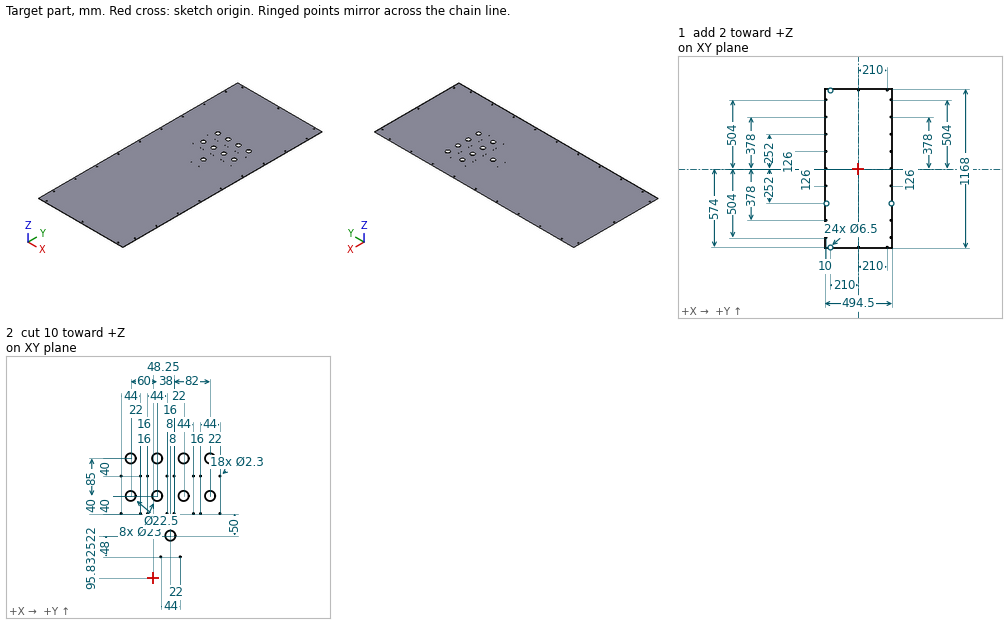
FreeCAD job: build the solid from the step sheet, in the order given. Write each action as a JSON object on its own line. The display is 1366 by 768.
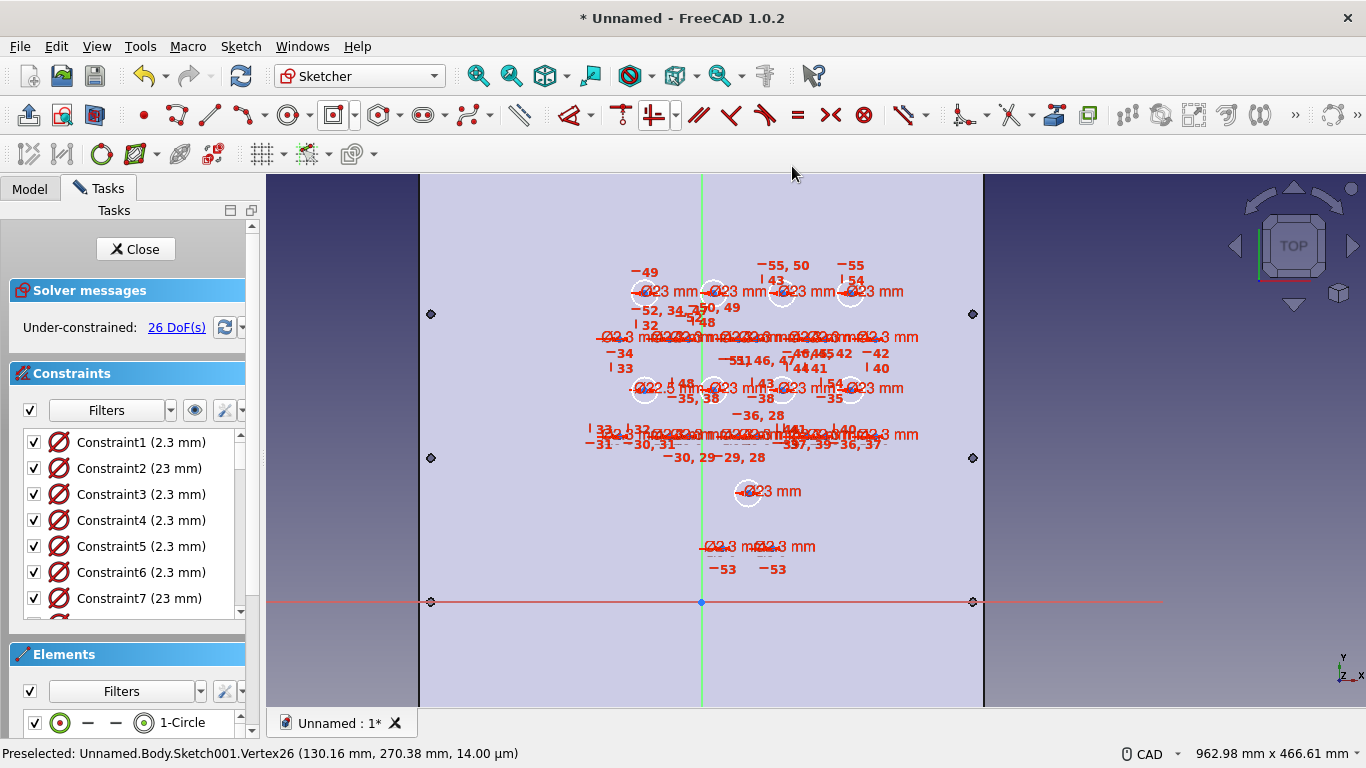
{"action": "left_click", "coordinate": [568, 116]}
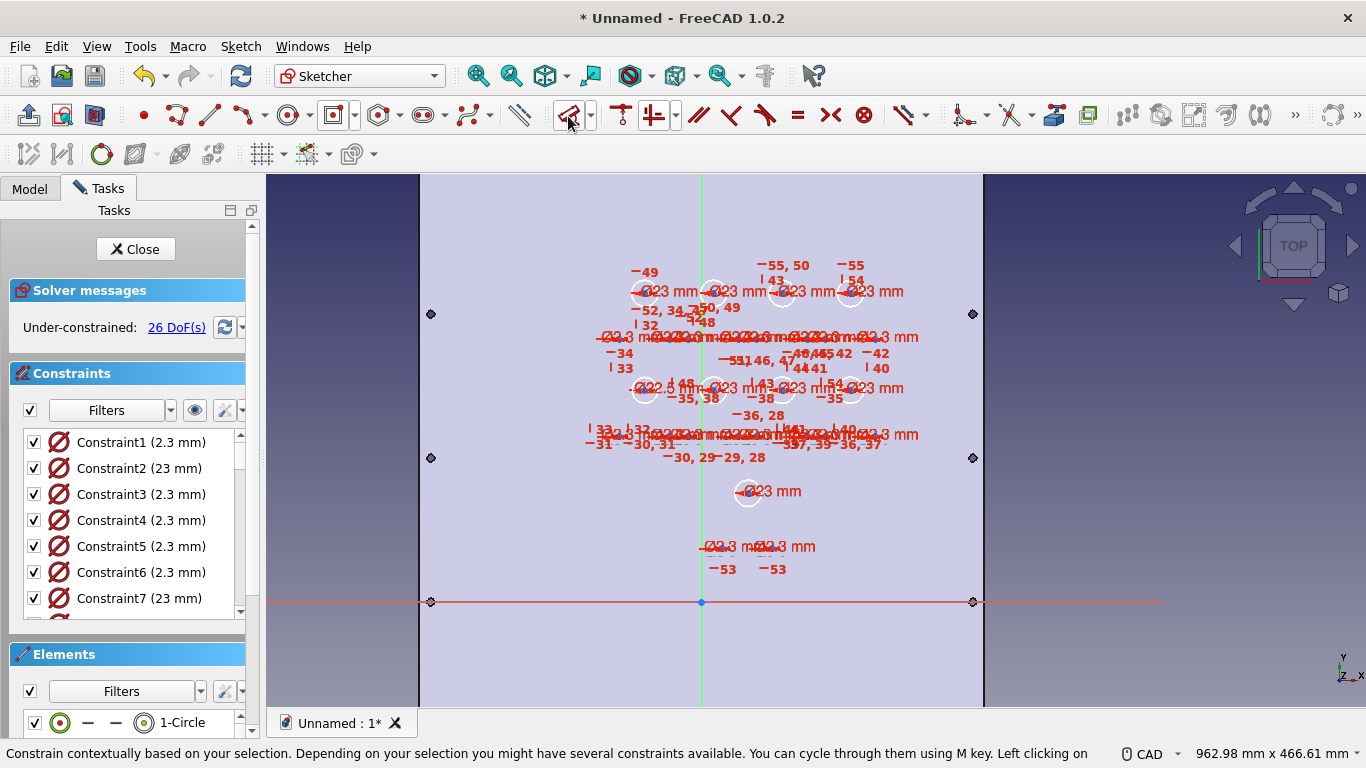
{"action": "scroll", "coordinate": [757, 437], "scroll_direction": "up", "scroll_amount": 8}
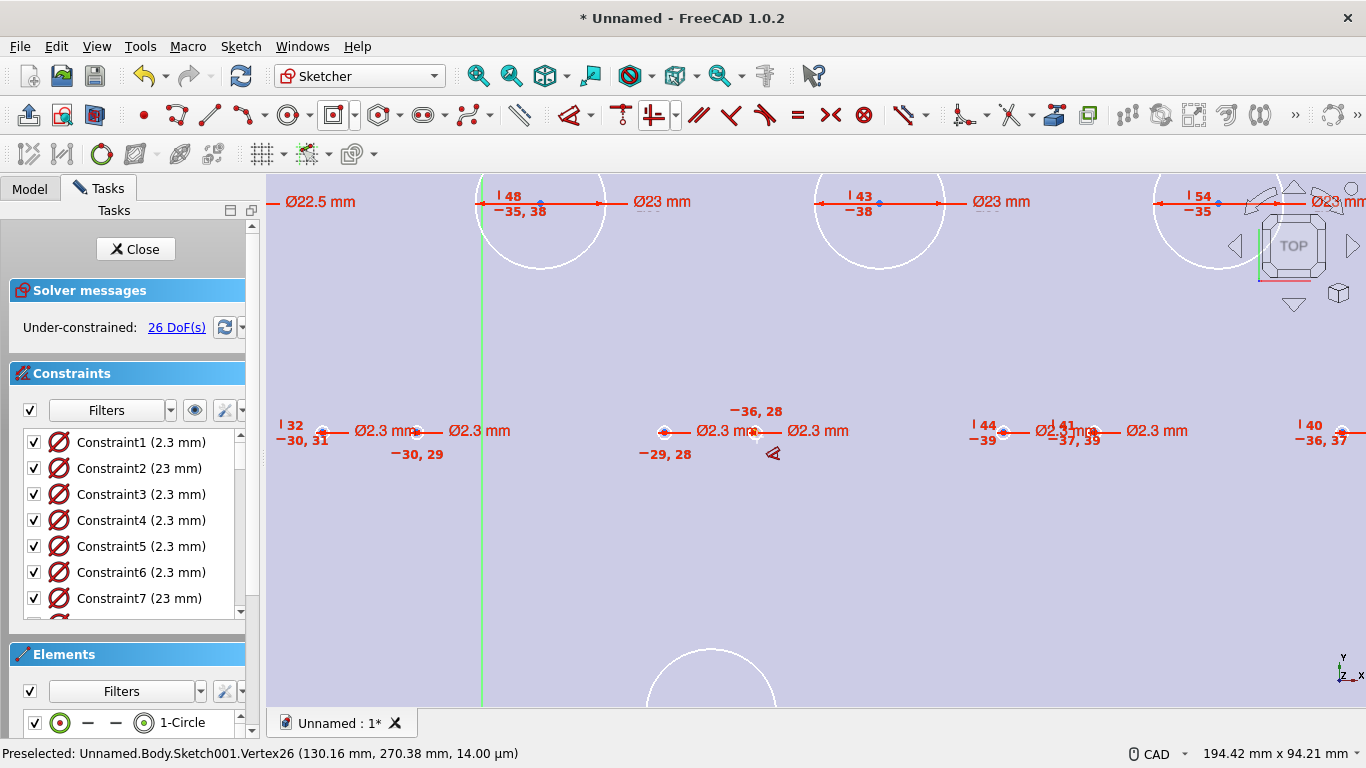
{"action": "left_click", "coordinate": [755, 433]}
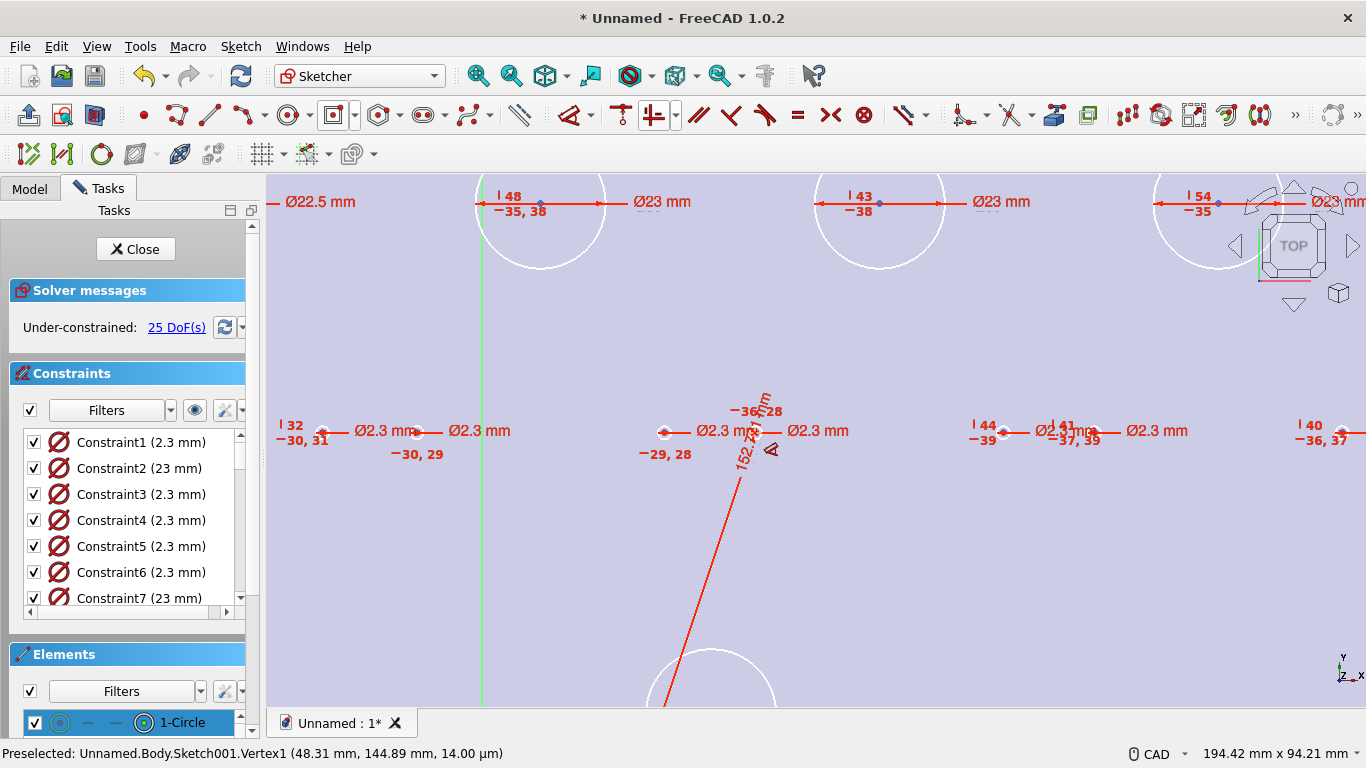
{"action": "scroll", "coordinate": [757, 437], "scroll_direction": "down", "scroll_amount": 8}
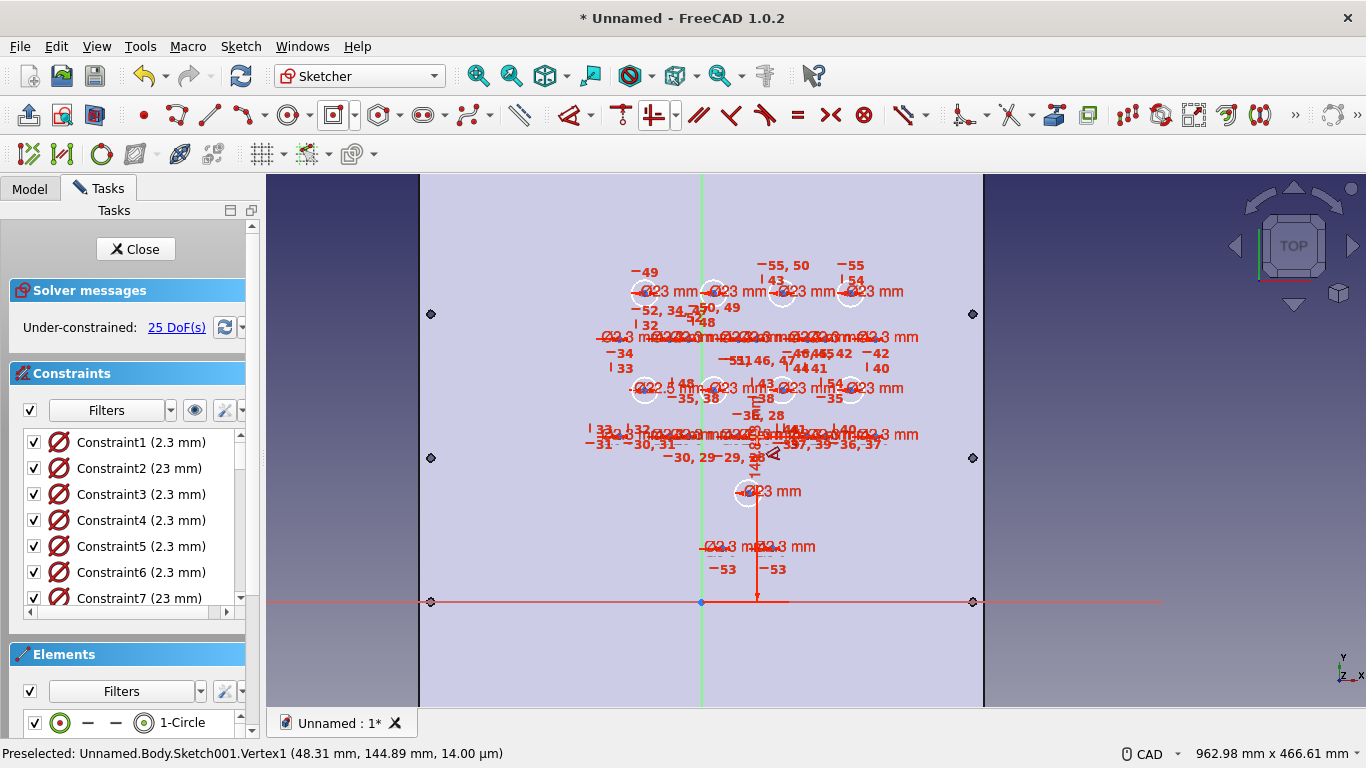
{"action": "scroll", "coordinate": [748, 493], "scroll_direction": "up", "scroll_amount": 8}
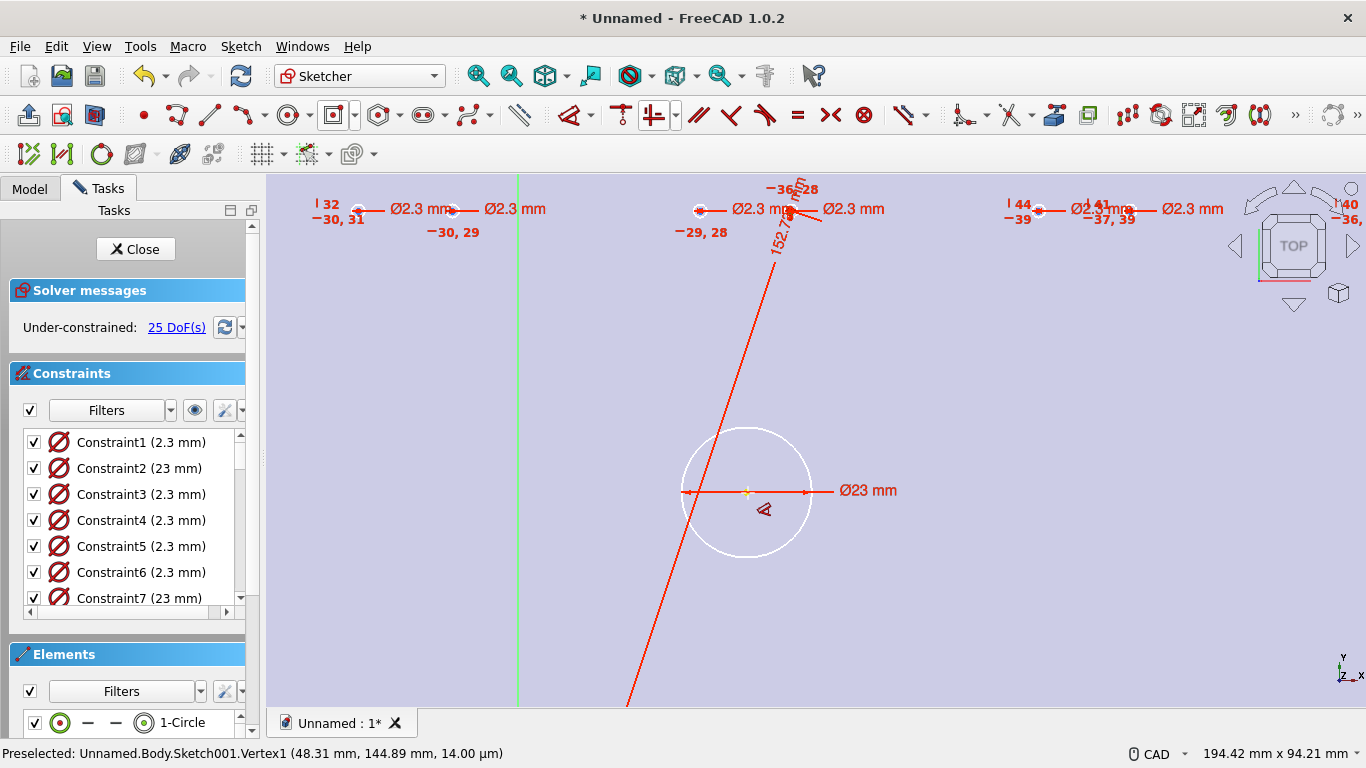
{"action": "left_click", "coordinate": [747, 492]}
{"action": "left_click", "coordinate": [769, 526]}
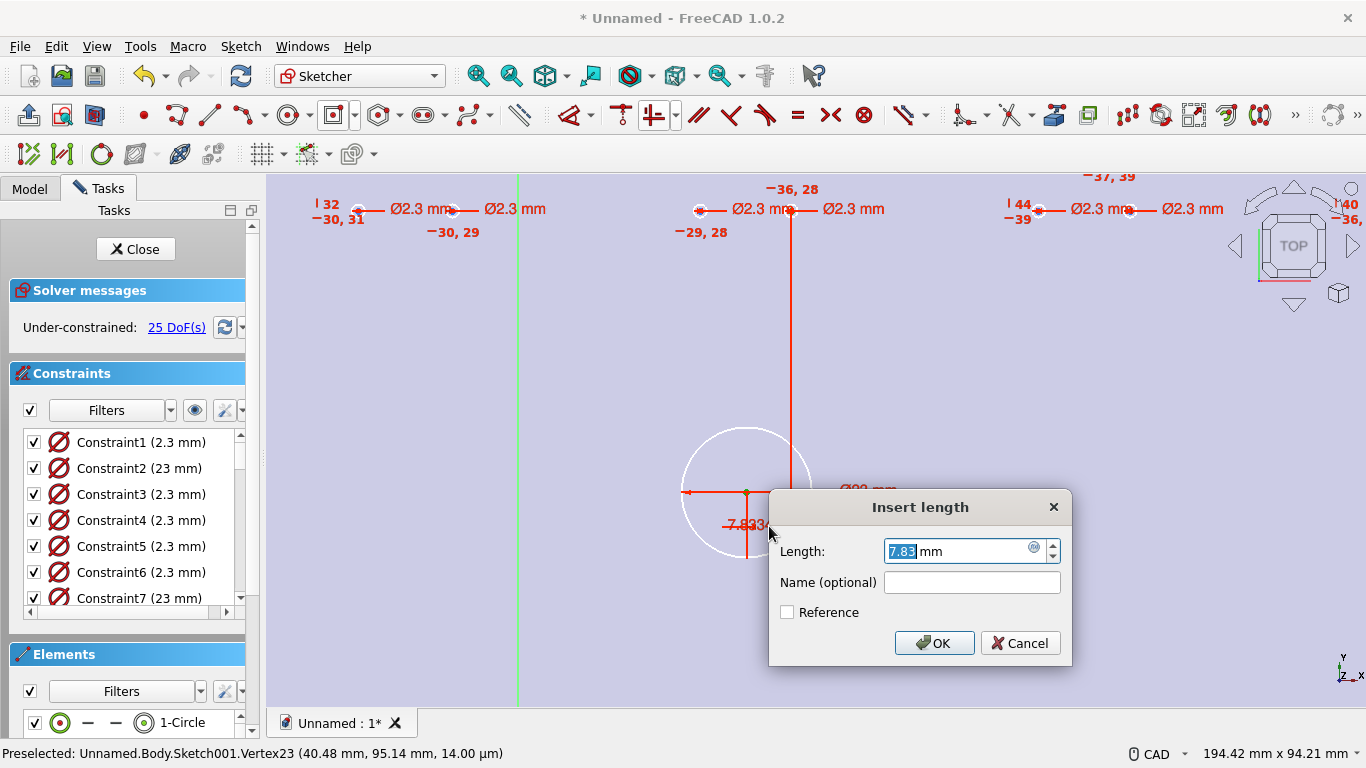
{"action": "type", "text": "8"}
{"action": "key", "text": "Return"}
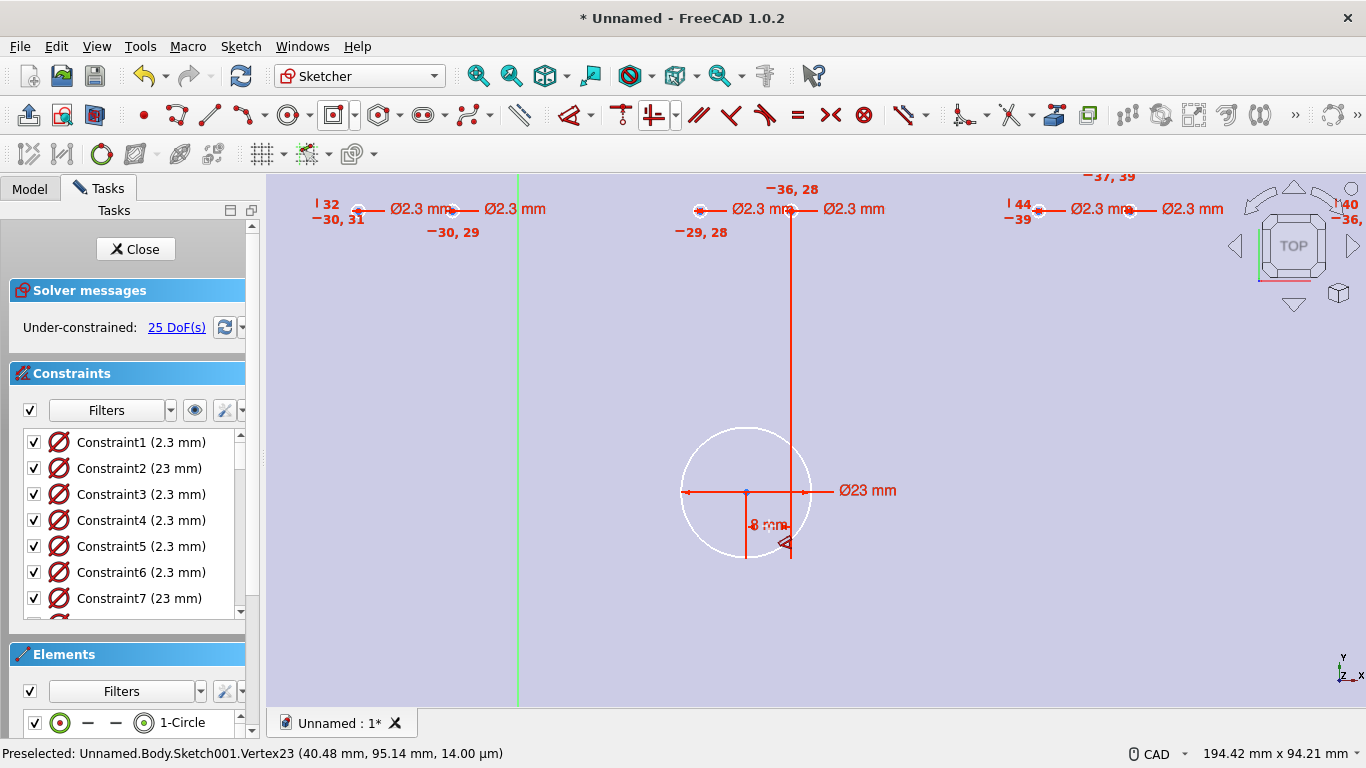
{"action": "left_click", "coordinate": [700, 211]}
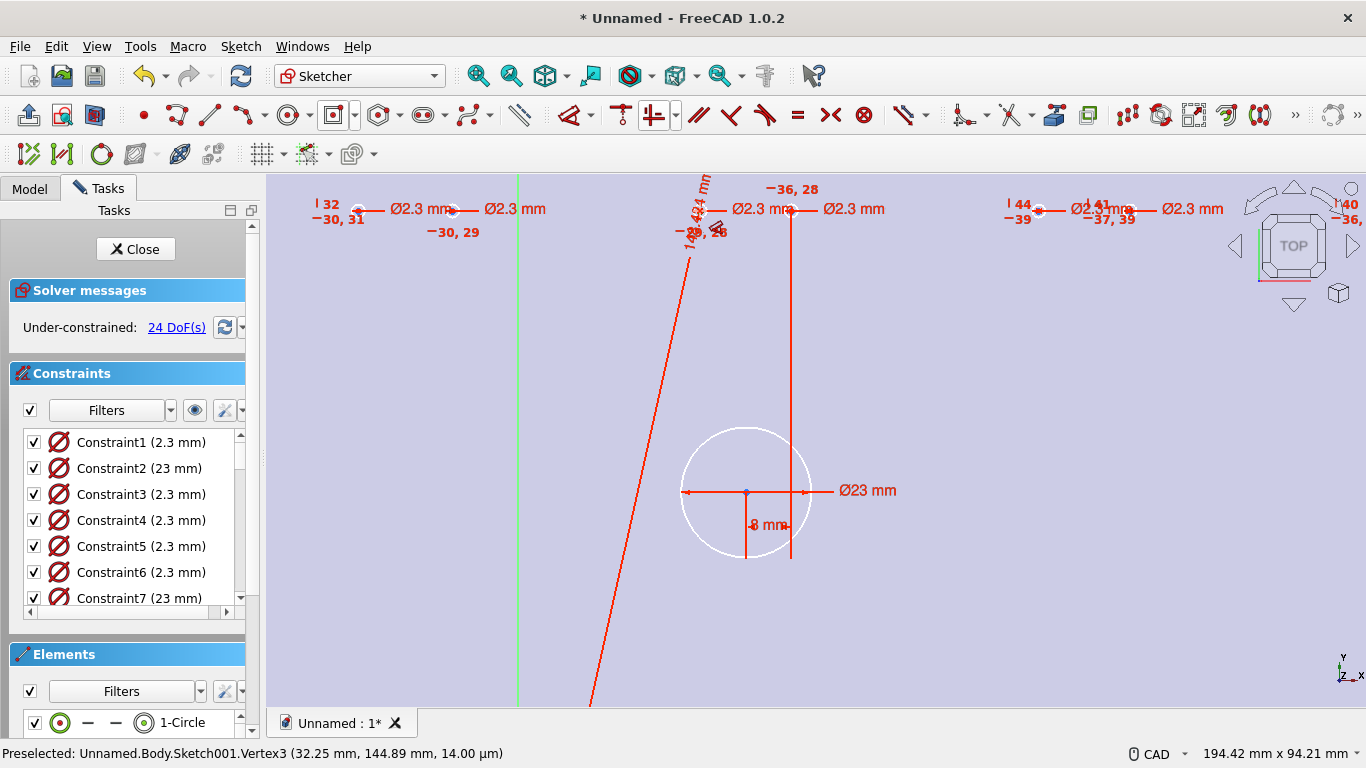
{"action": "left_click", "coordinate": [746, 492]}
{"action": "left_click", "coordinate": [723, 574]}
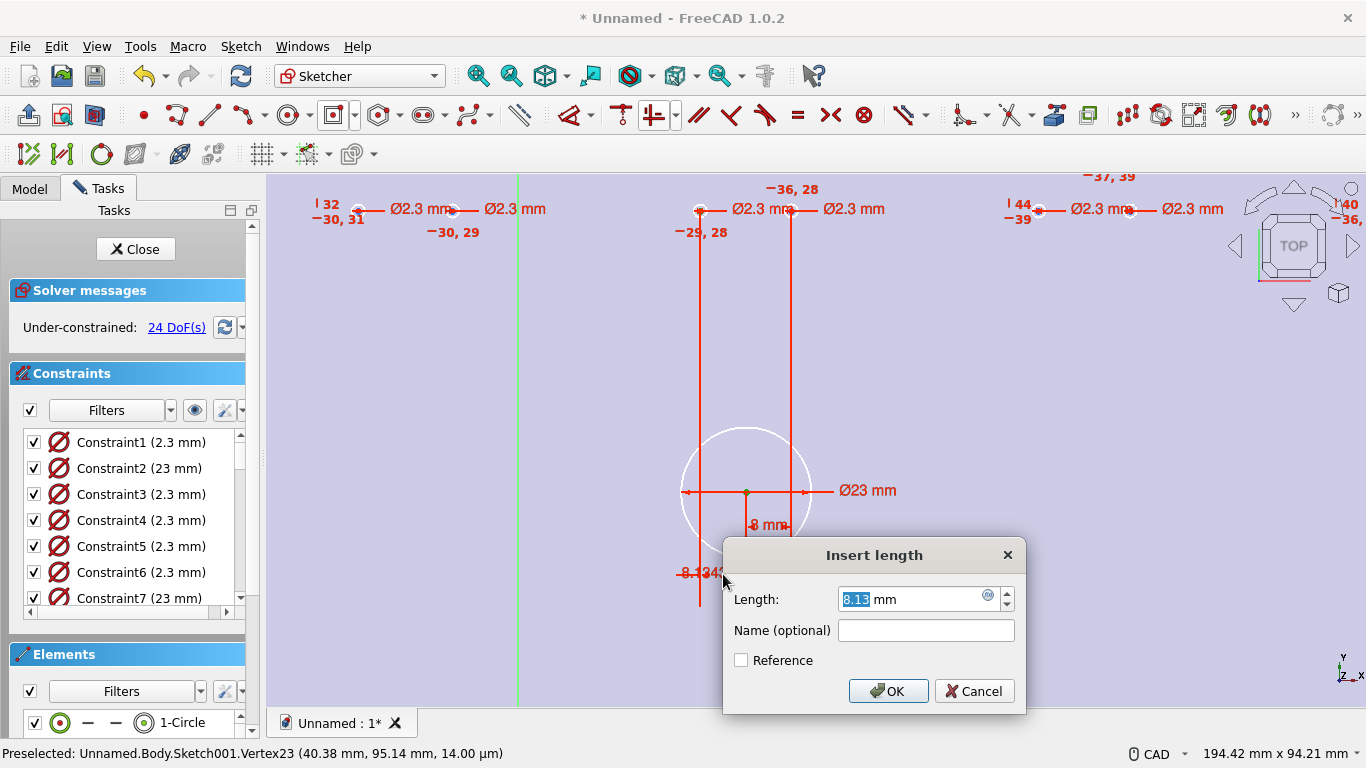
{"action": "type", "text": "8"}
{"action": "key", "text": "Return"}